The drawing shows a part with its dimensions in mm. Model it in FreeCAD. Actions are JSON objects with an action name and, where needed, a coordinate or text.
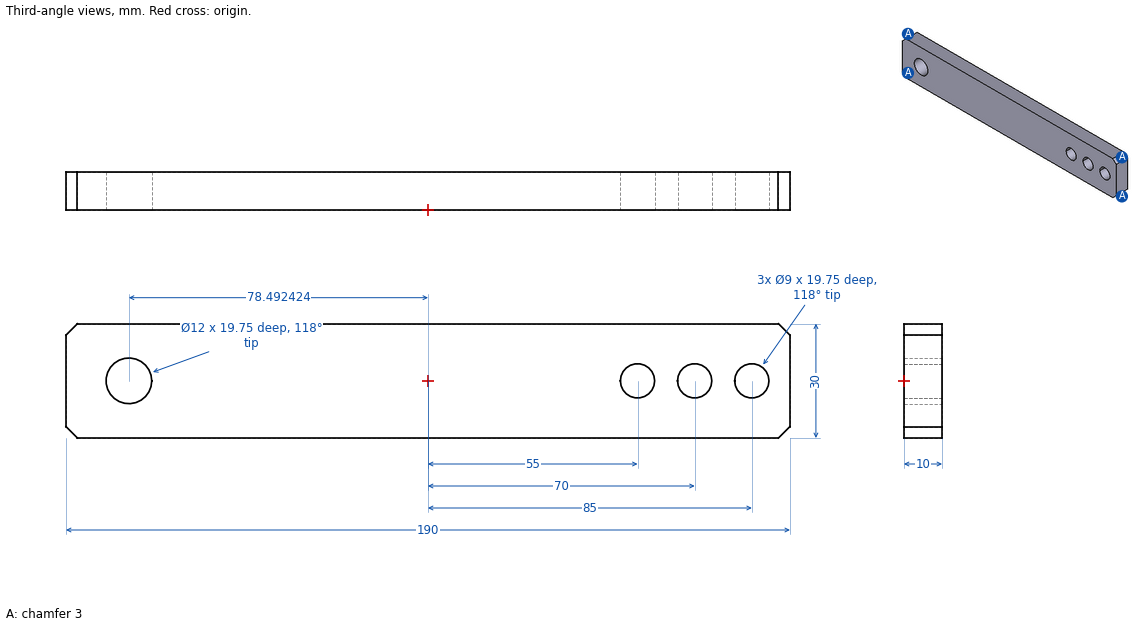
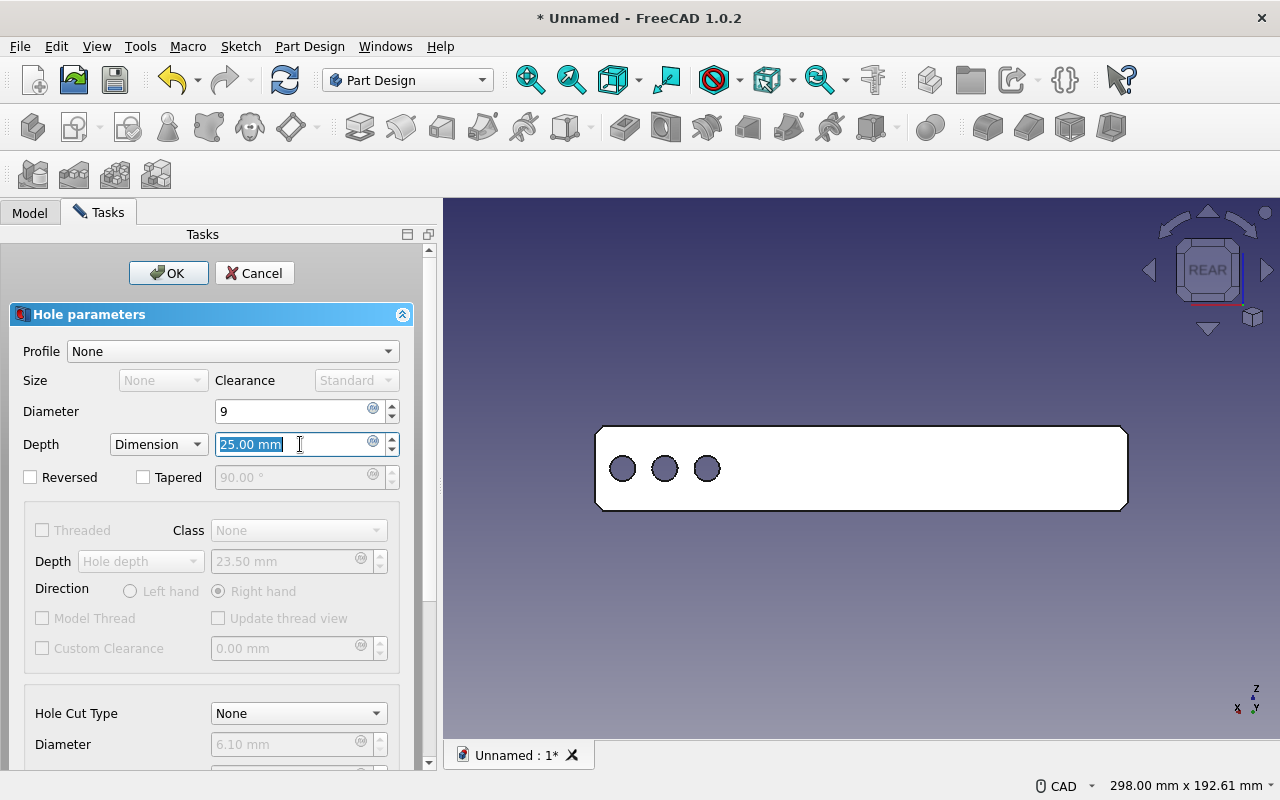
{"action": "type", "text": "19.75"}
{"action": "key", "text": "Tab"}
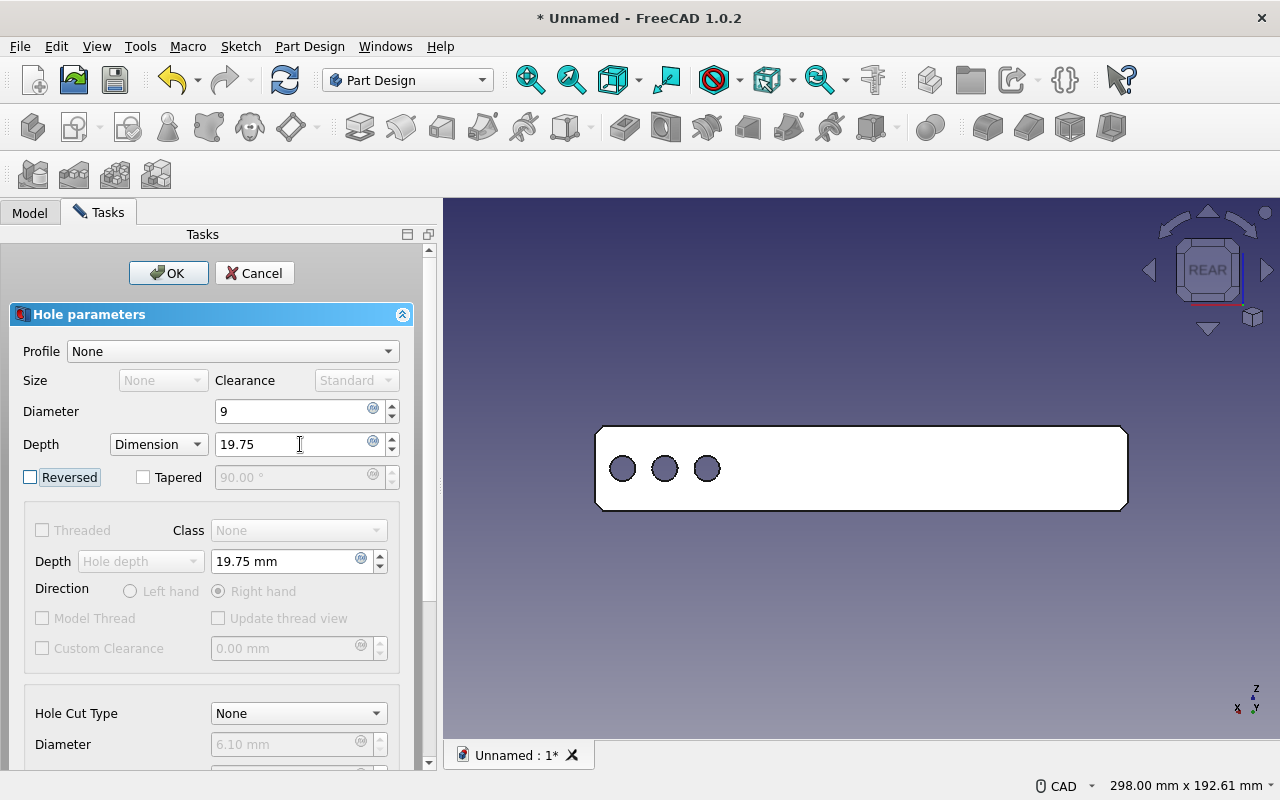
{"action": "left_click", "coordinate": [169, 273]}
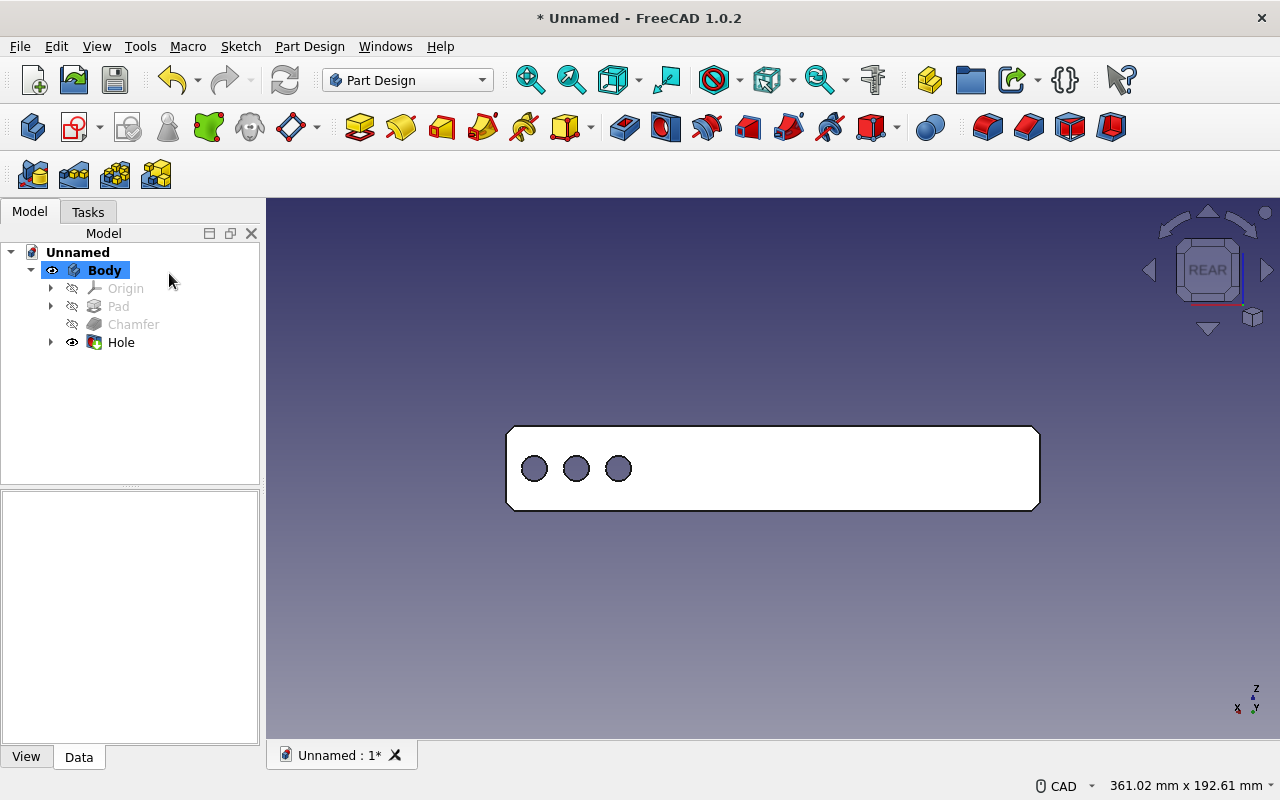
{"action": "left_click", "coordinate": [74, 128]}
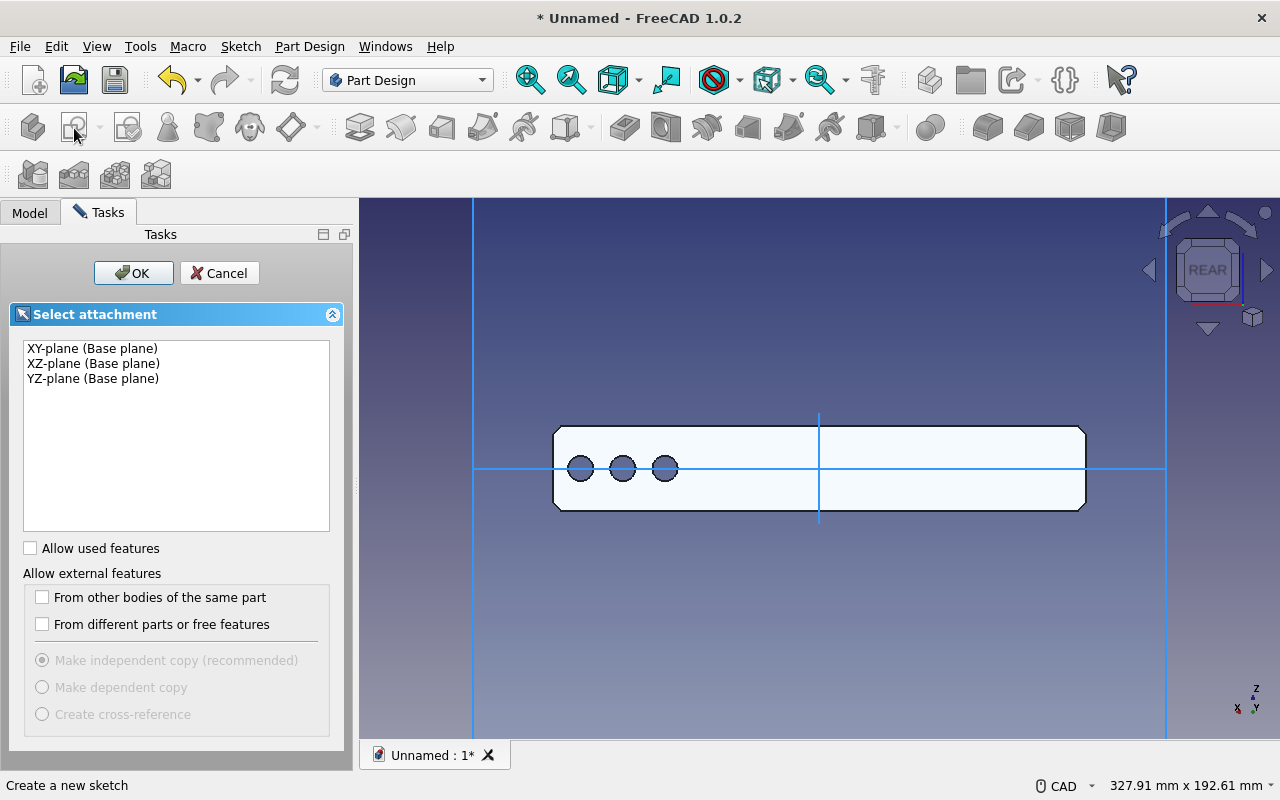
{"action": "left_click", "coordinate": [84, 364]}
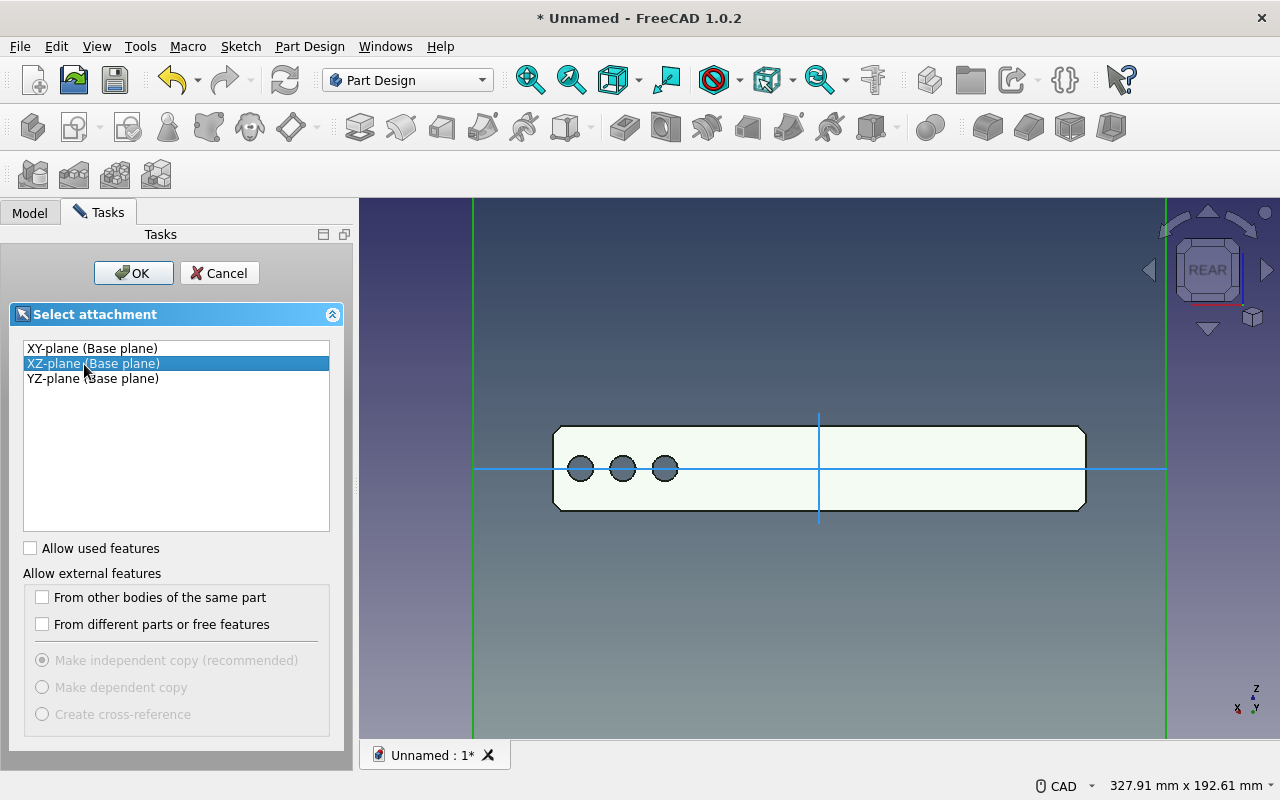
{"action": "left_click", "coordinate": [134, 273]}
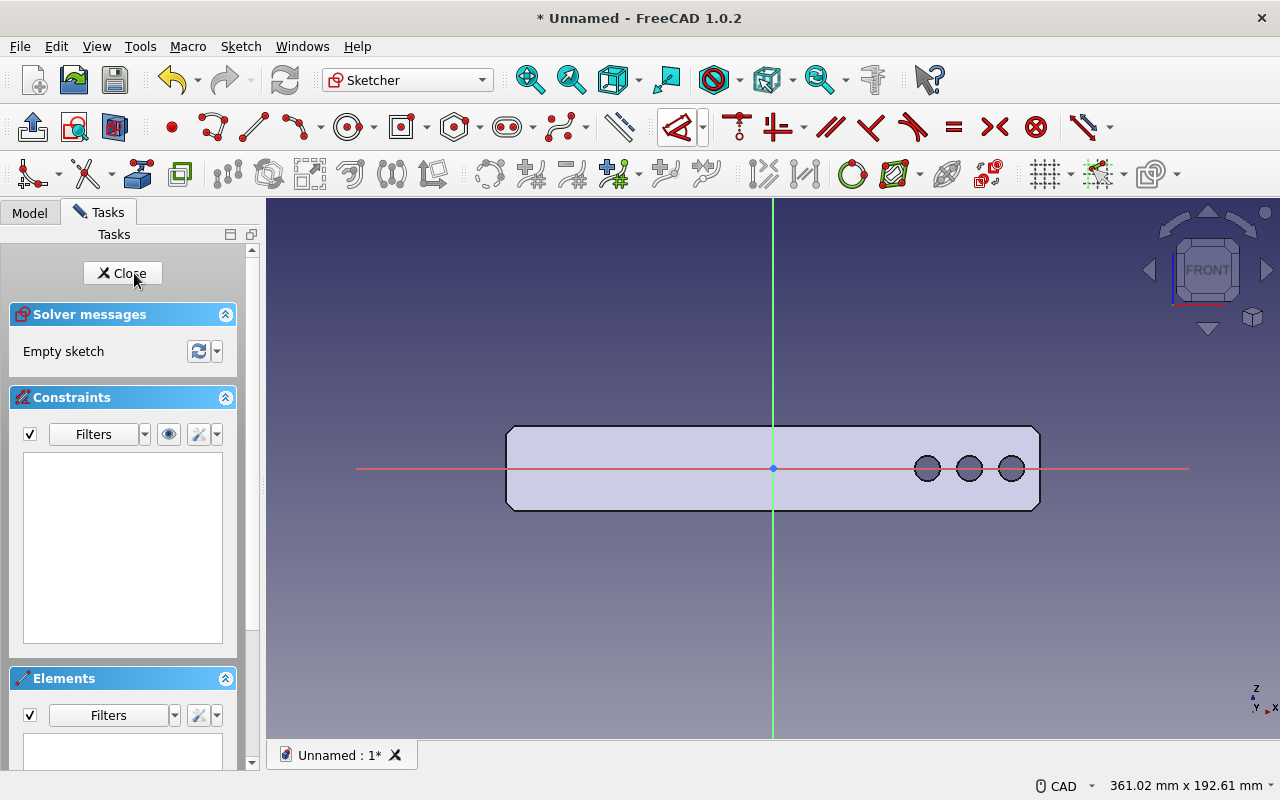
{"action": "scroll", "coordinate": [537, 469], "scroll_direction": "up", "scroll_amount": 12}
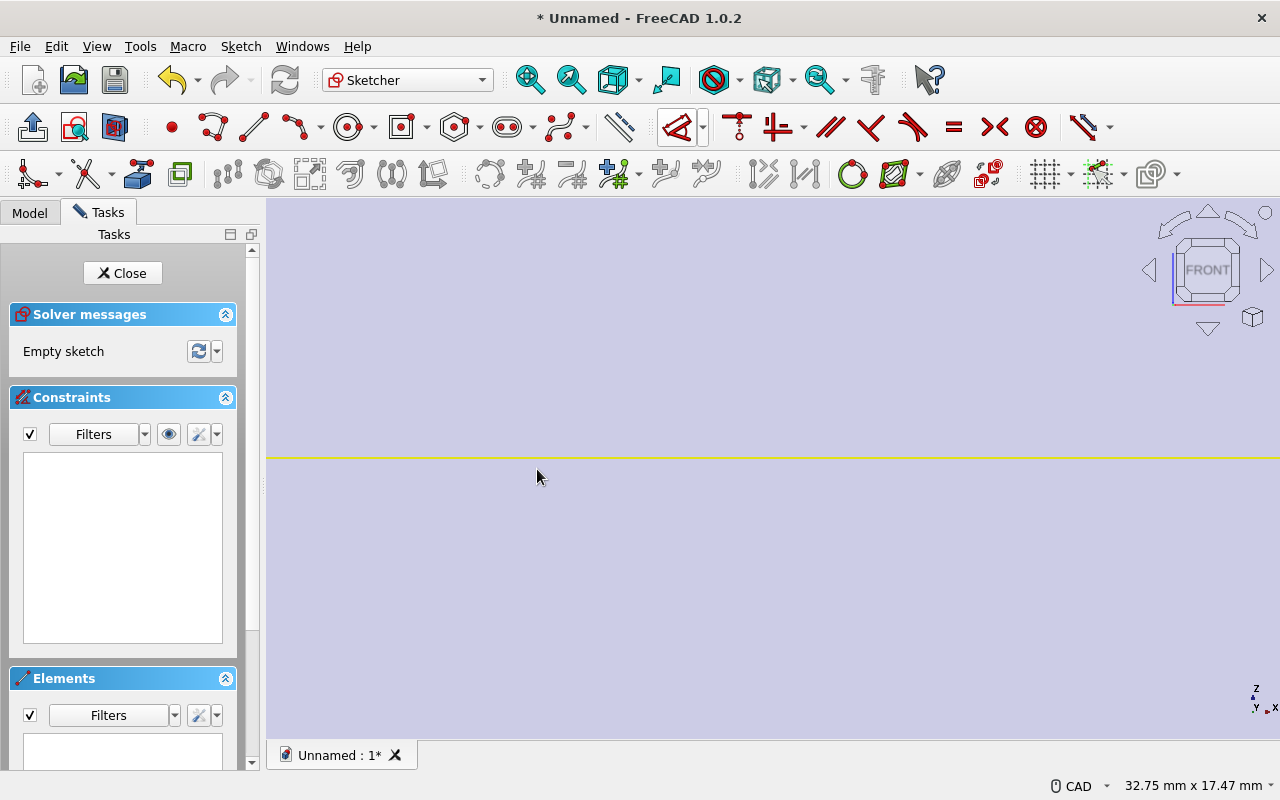
{"action": "left_click", "coordinate": [348, 128]}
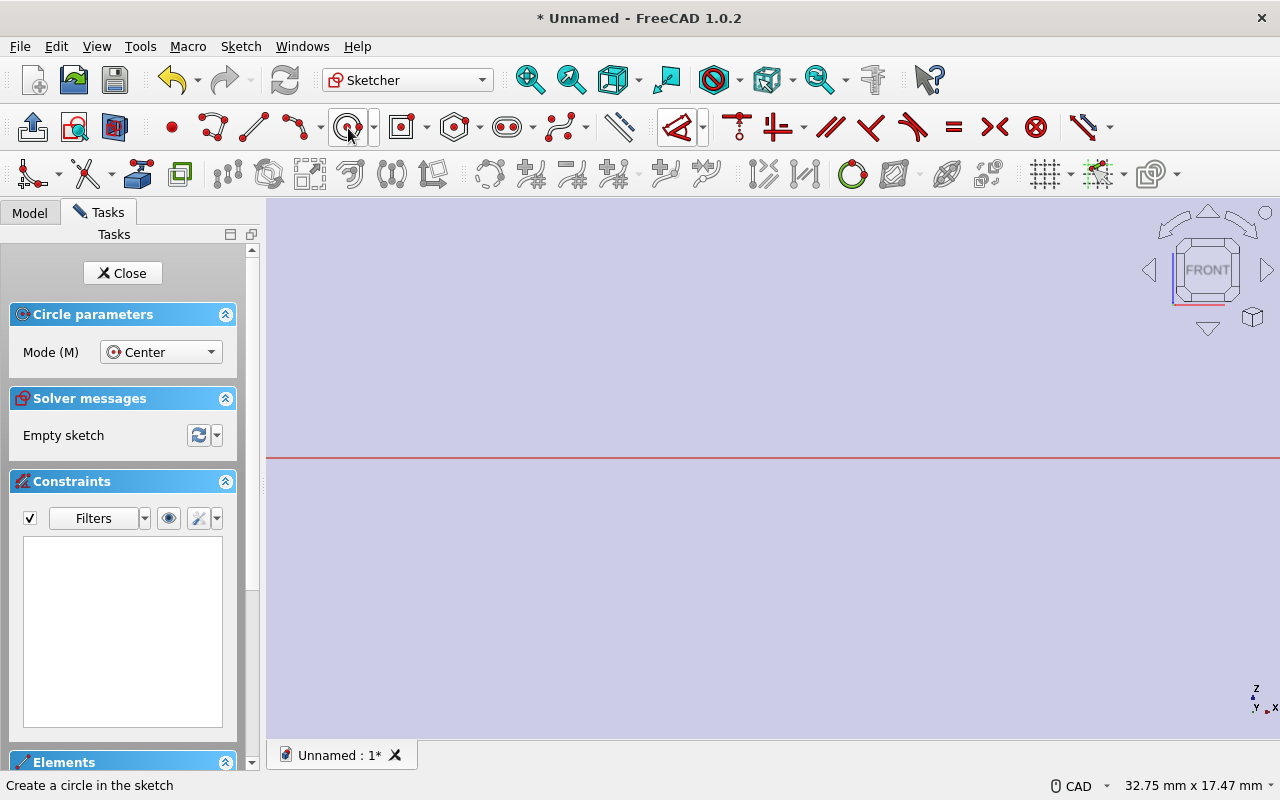
{"action": "left_click", "coordinate": [706, 458]}
{"action": "mouse_move", "coordinate": [837, 327]}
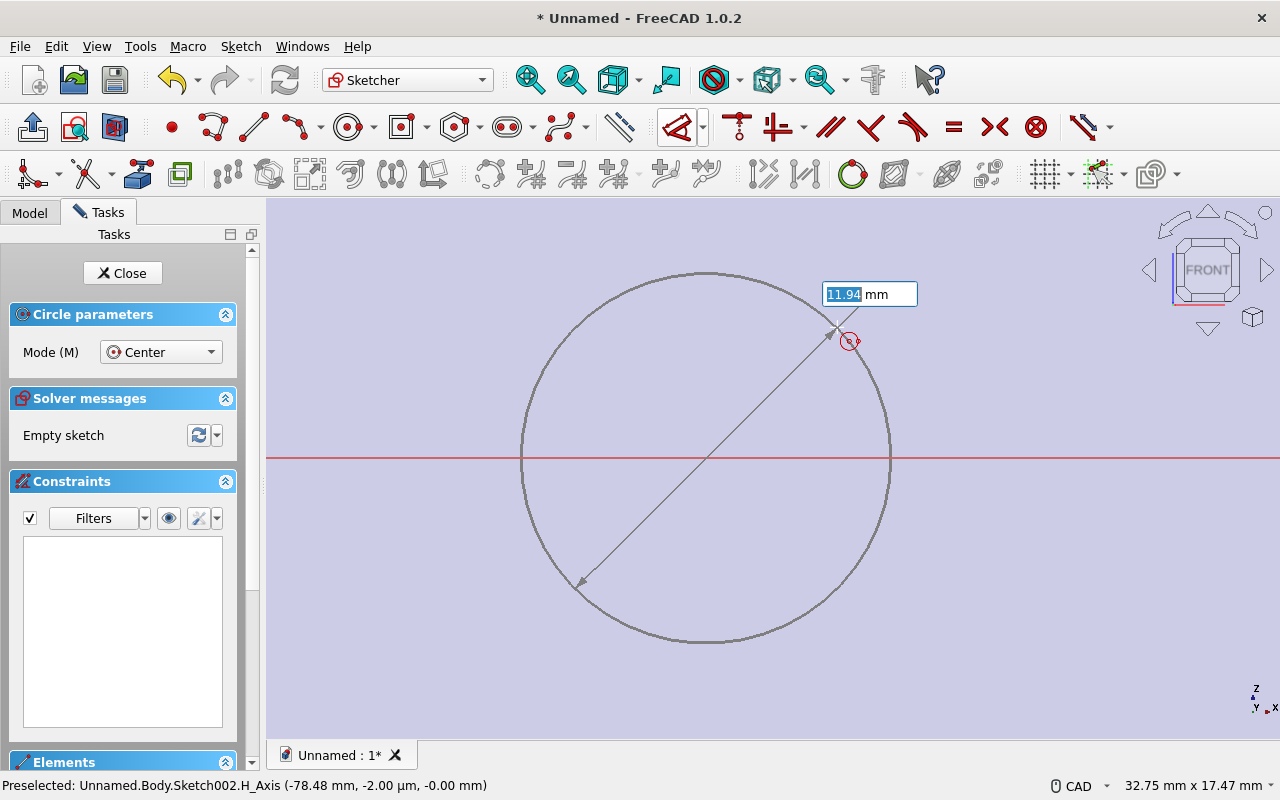
{"action": "type", "text": "12"}
{"action": "key", "text": "Return"}
{"action": "key", "text": "Escape"}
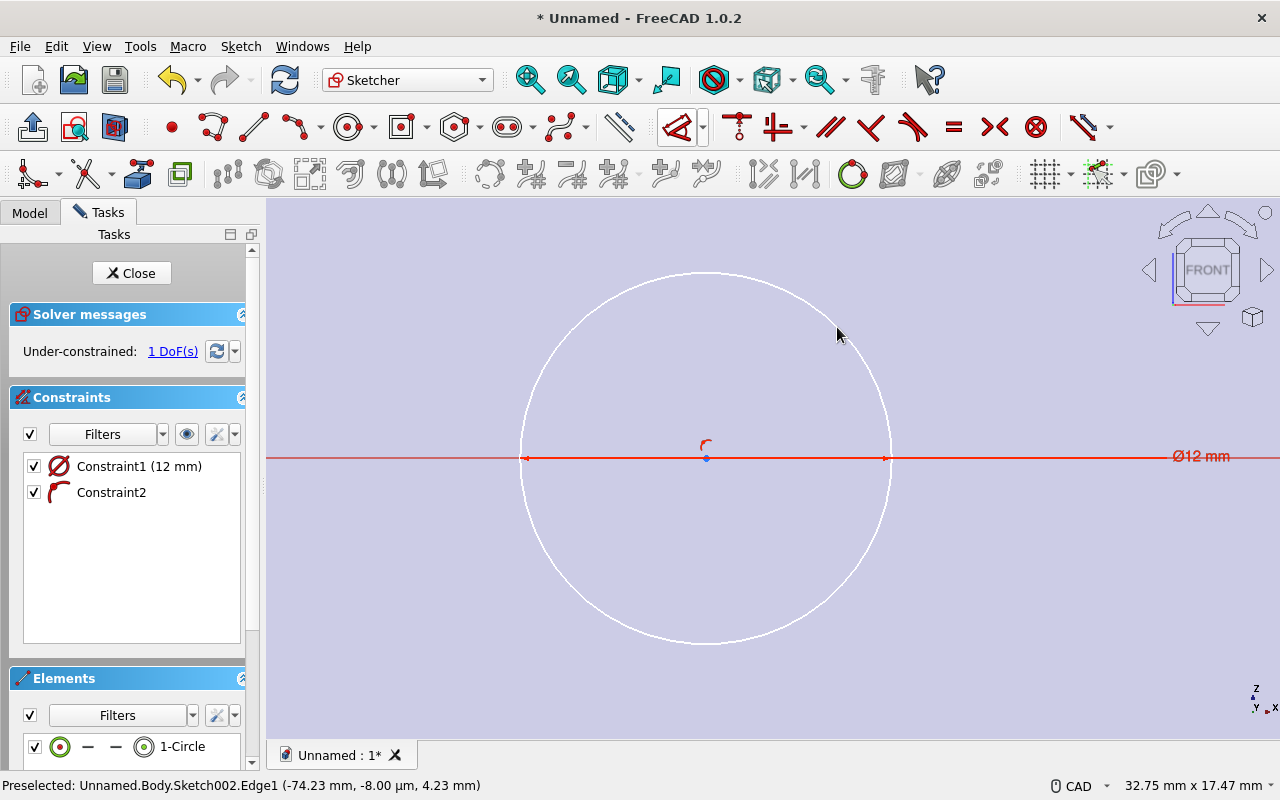
{"action": "left_click", "coordinate": [676, 128]}